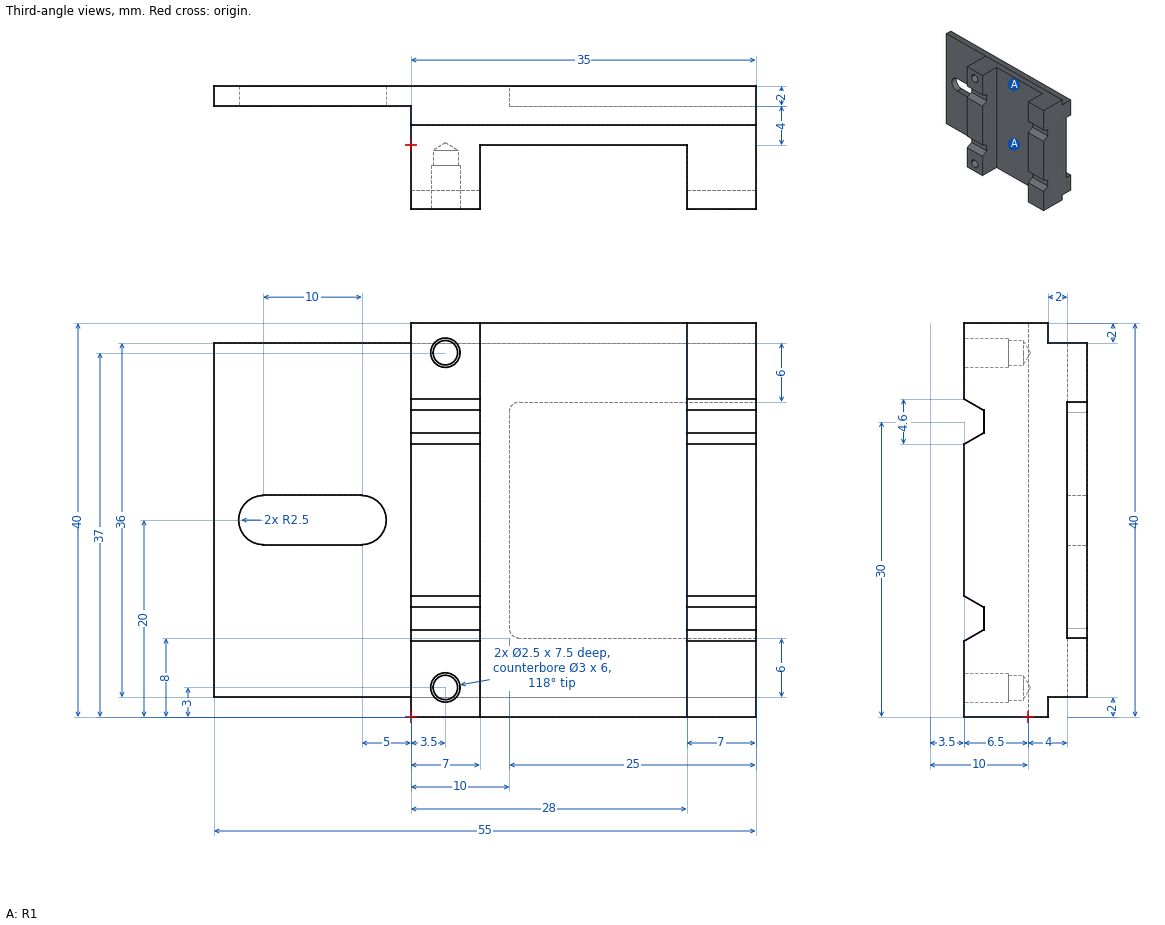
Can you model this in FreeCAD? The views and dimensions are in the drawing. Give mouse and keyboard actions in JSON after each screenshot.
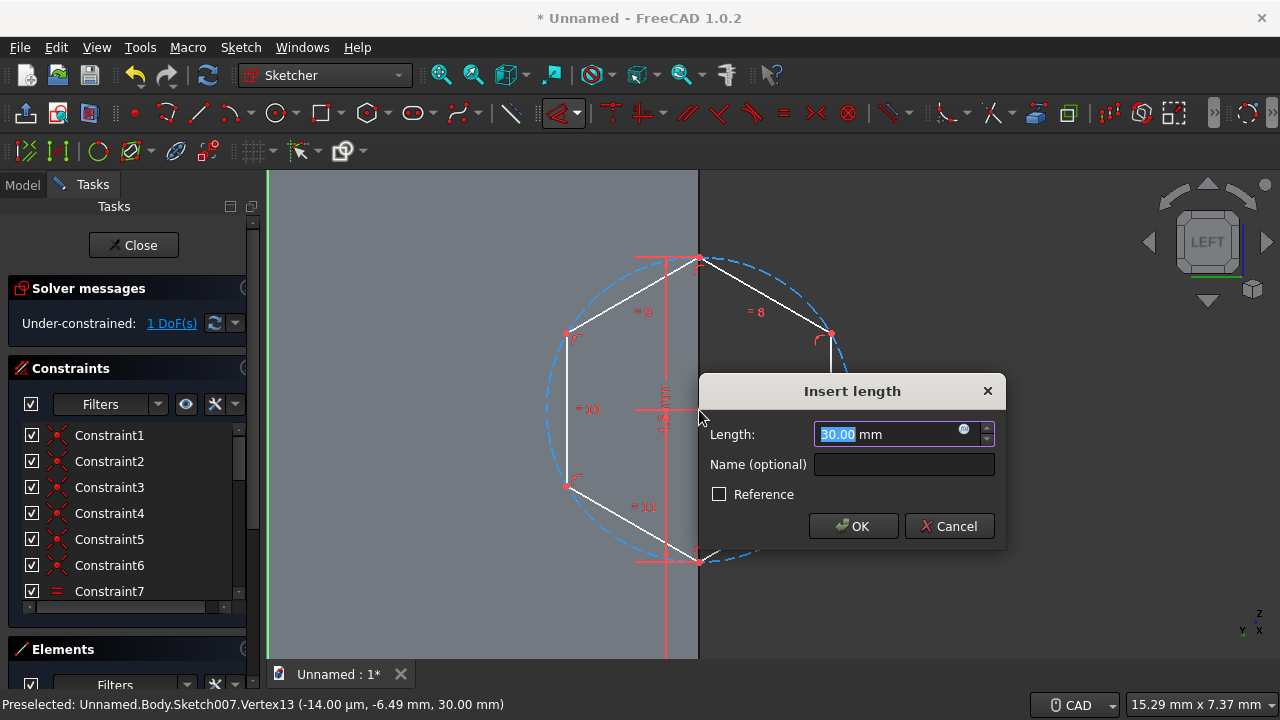
{"action": "type", "text": "30"}
{"action": "key", "text": "Return"}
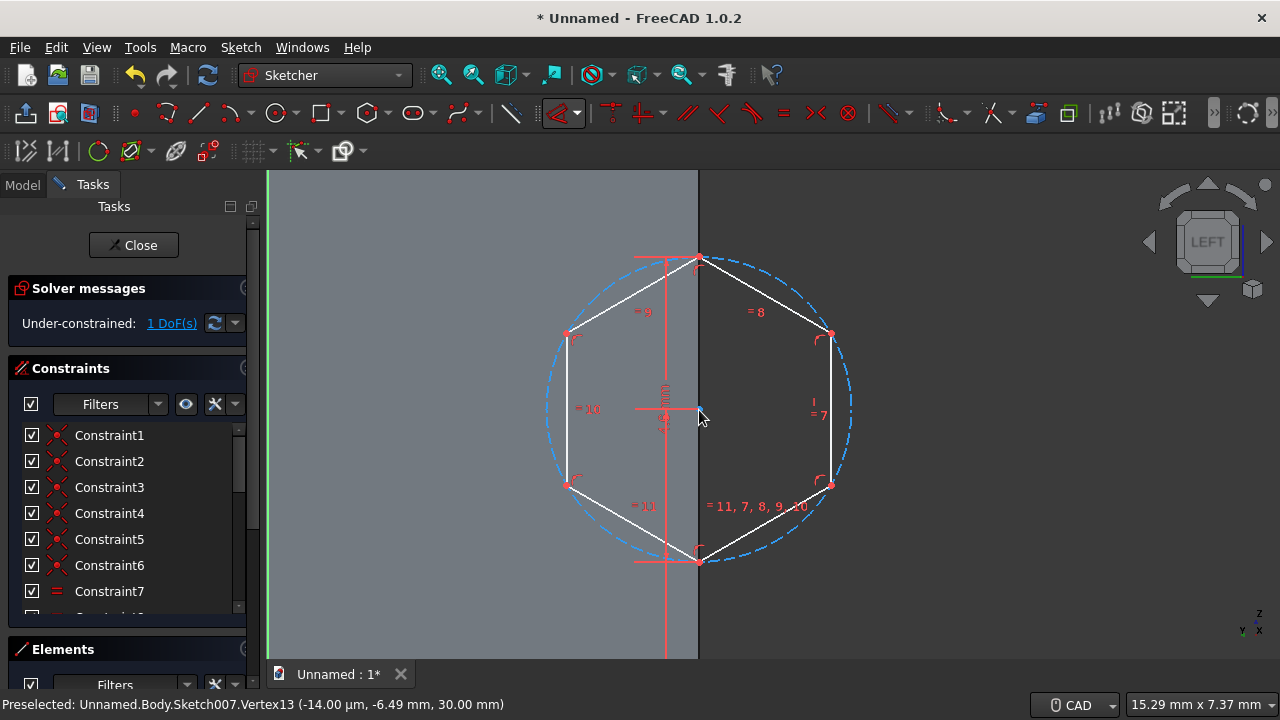
{"action": "left_click", "coordinate": [699, 409]}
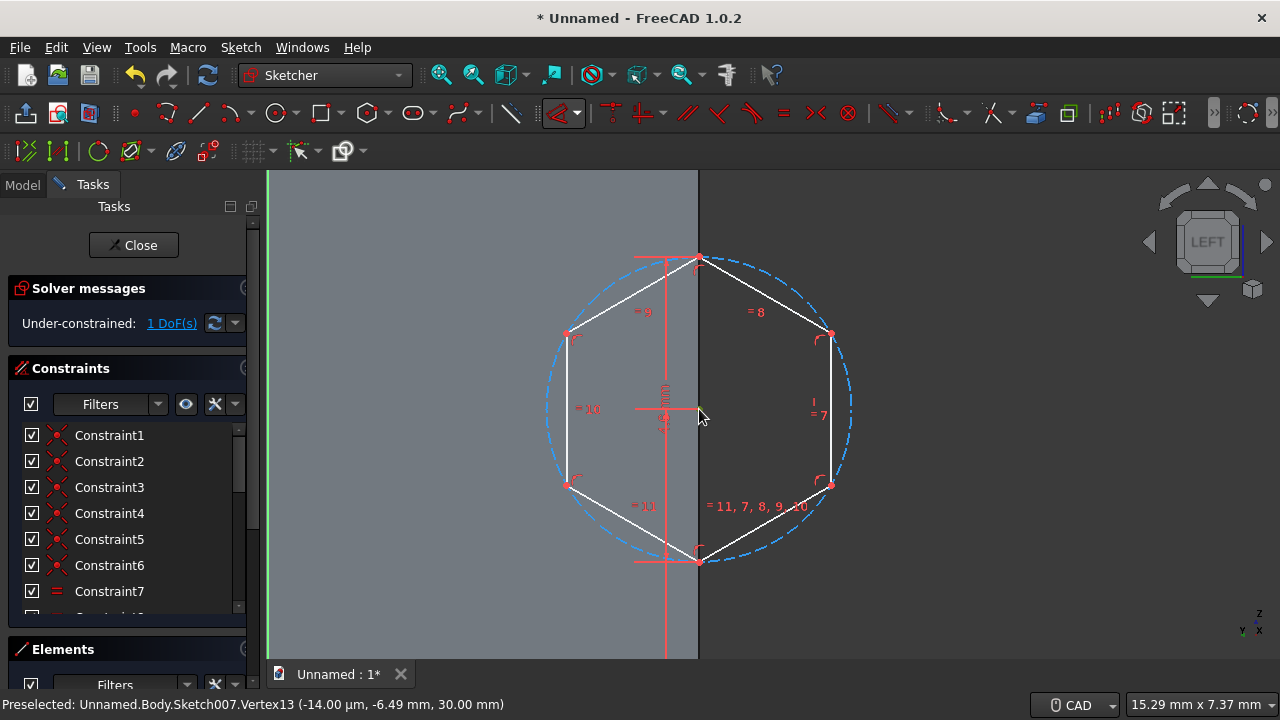
{"action": "key", "text": "l"}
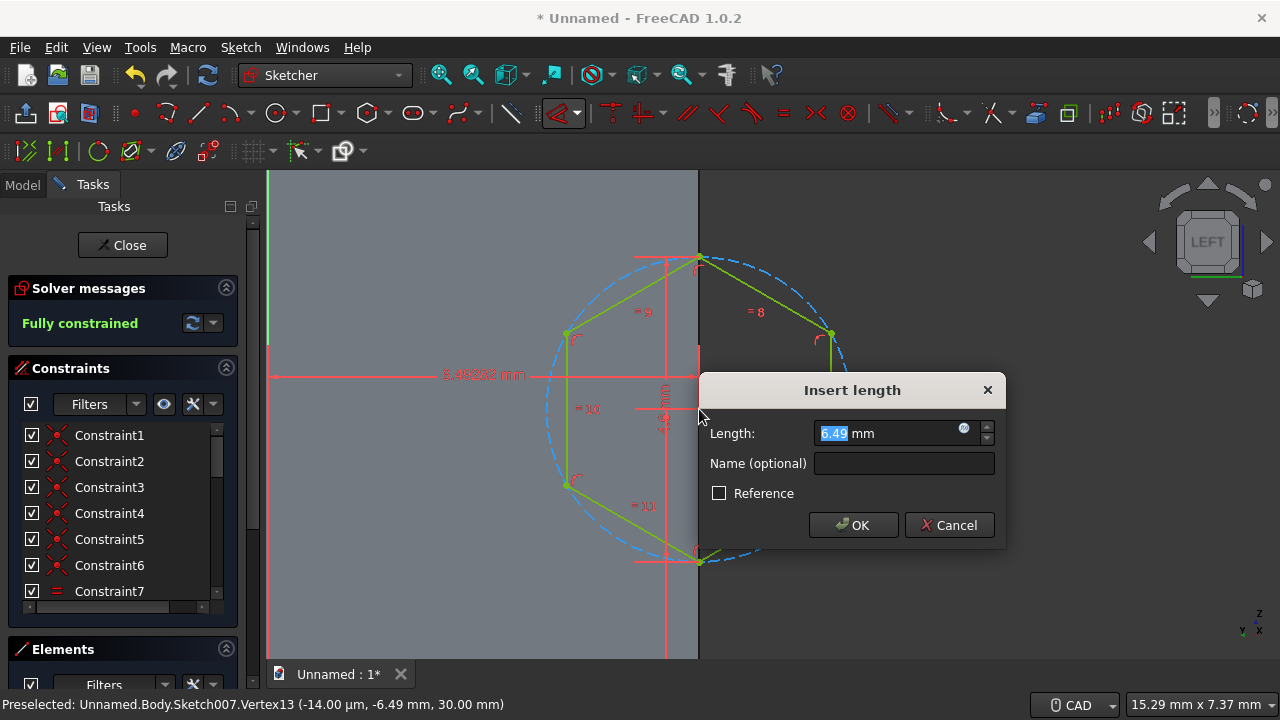
{"action": "type", "text": "6.5"}
{"action": "key", "text": "Return"}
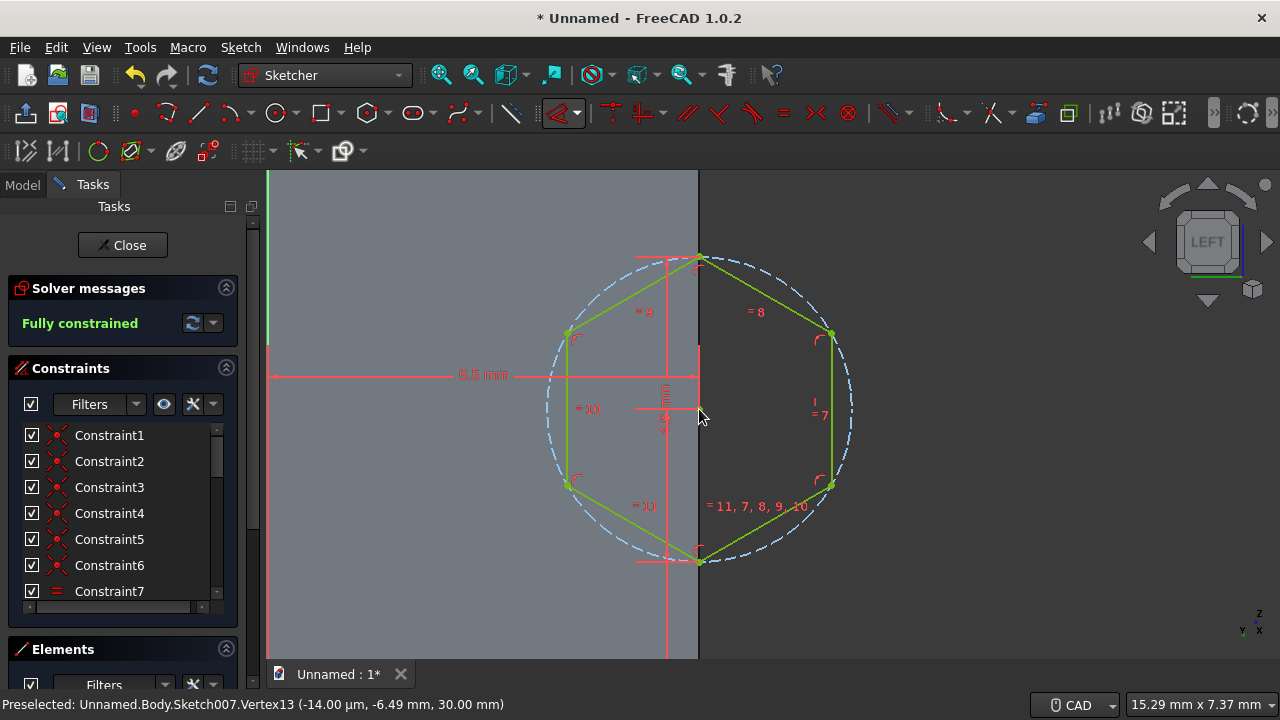
{"action": "left_click", "coordinate": [123, 245]}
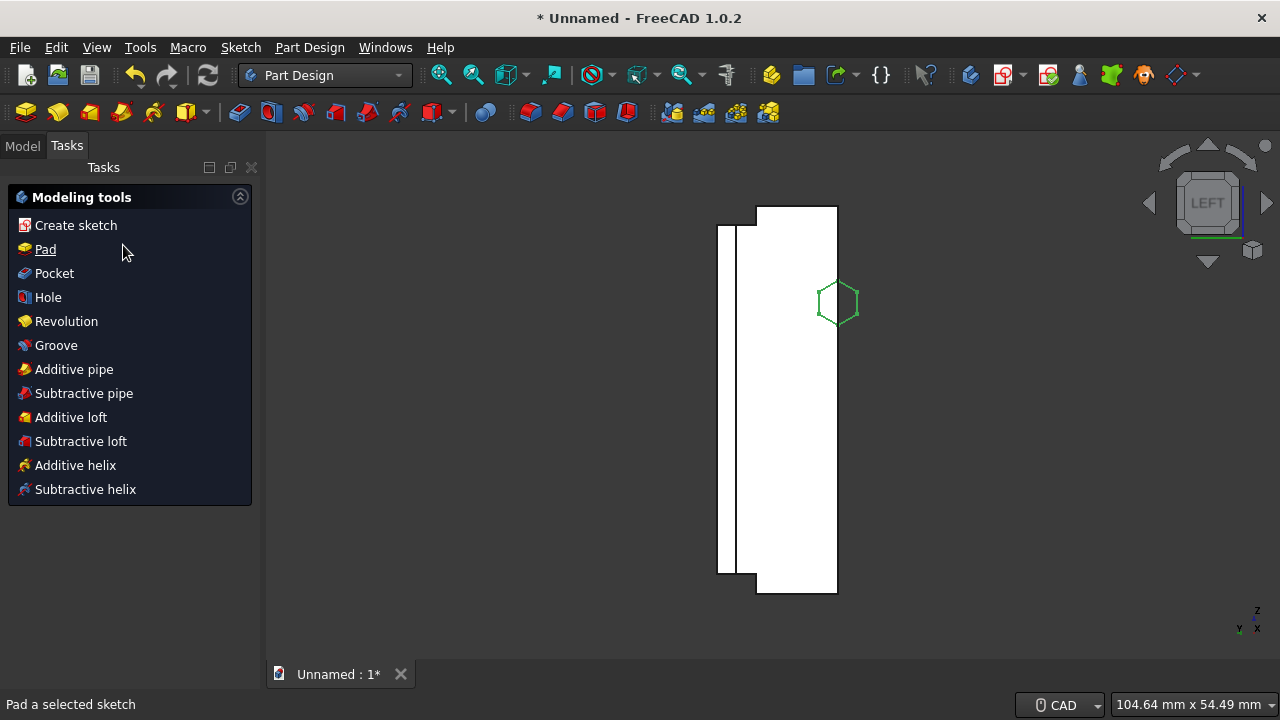
{"action": "left_click", "coordinate": [240, 112]}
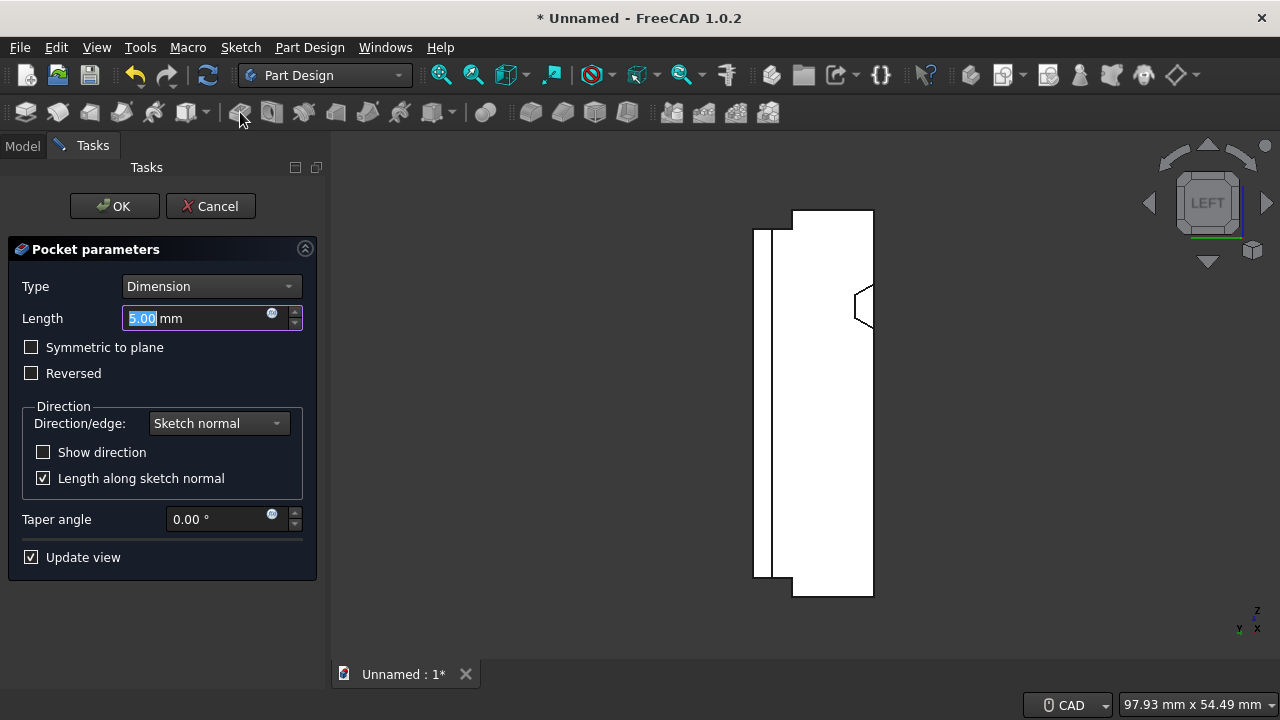
{"action": "left_click", "coordinate": [212, 286]}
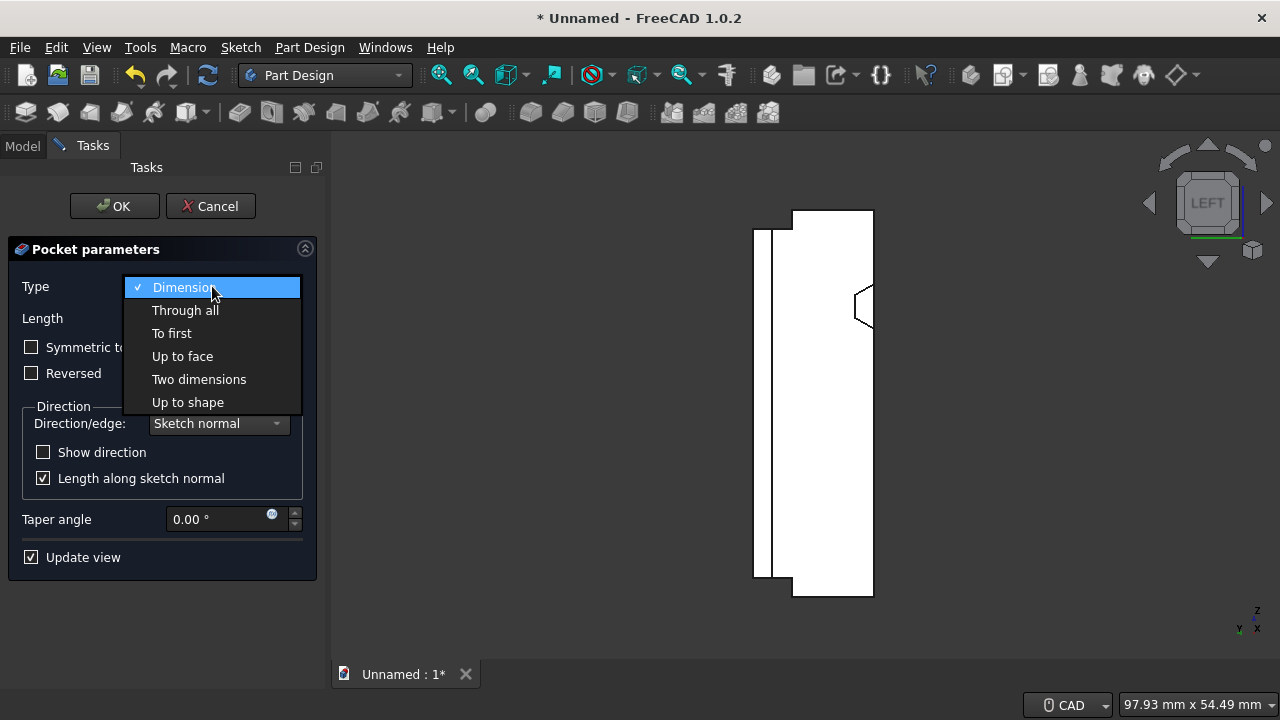
{"action": "left_click", "coordinate": [212, 310]}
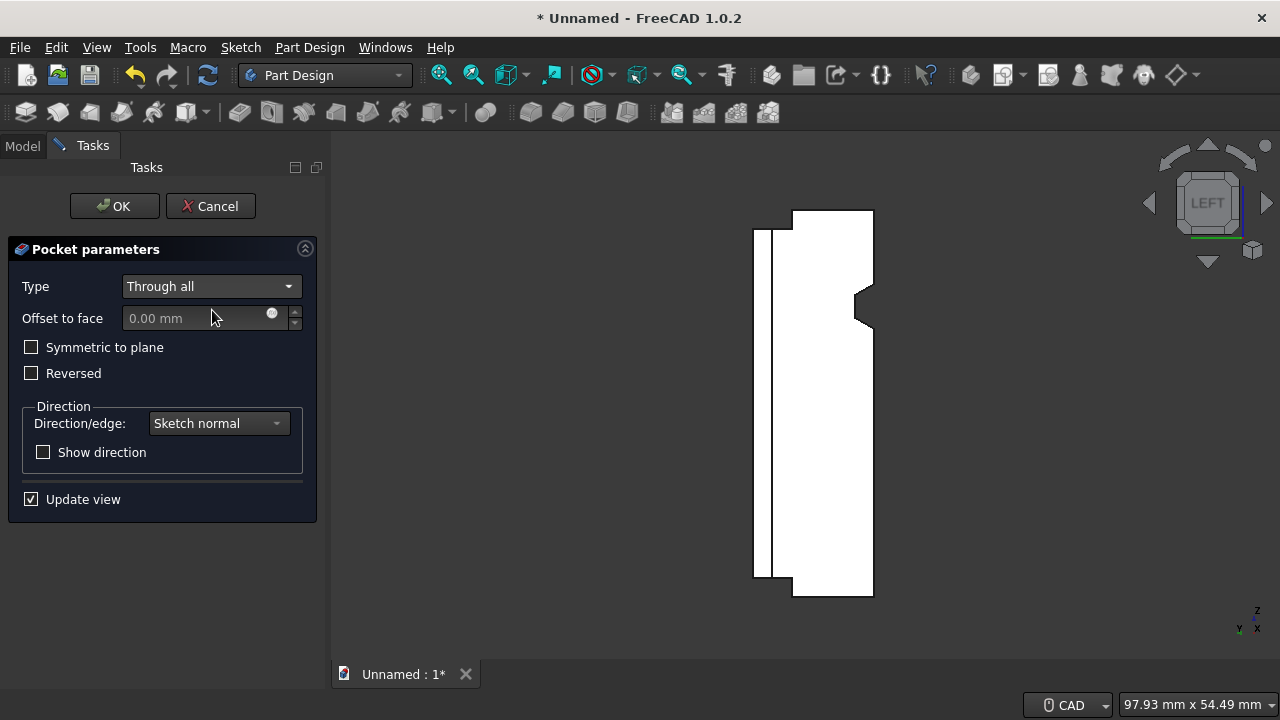
{"action": "left_click", "coordinate": [115, 206]}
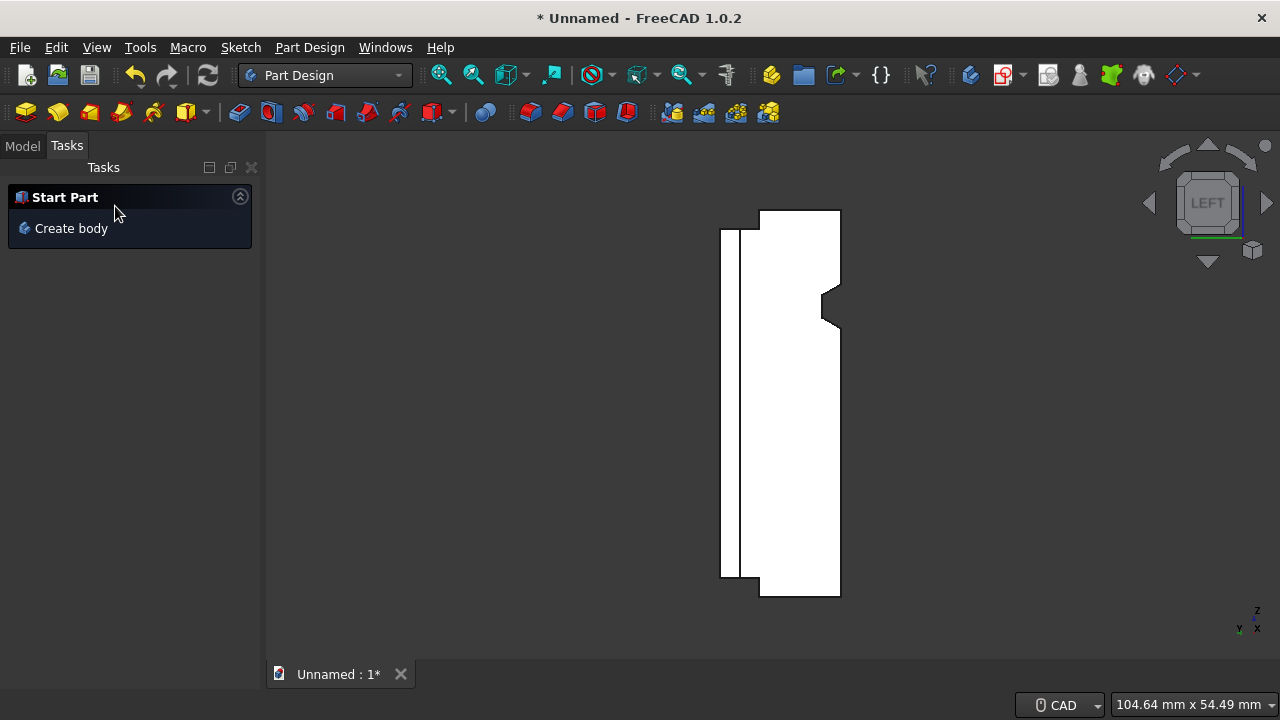
{"action": "left_click", "coordinate": [23, 145]}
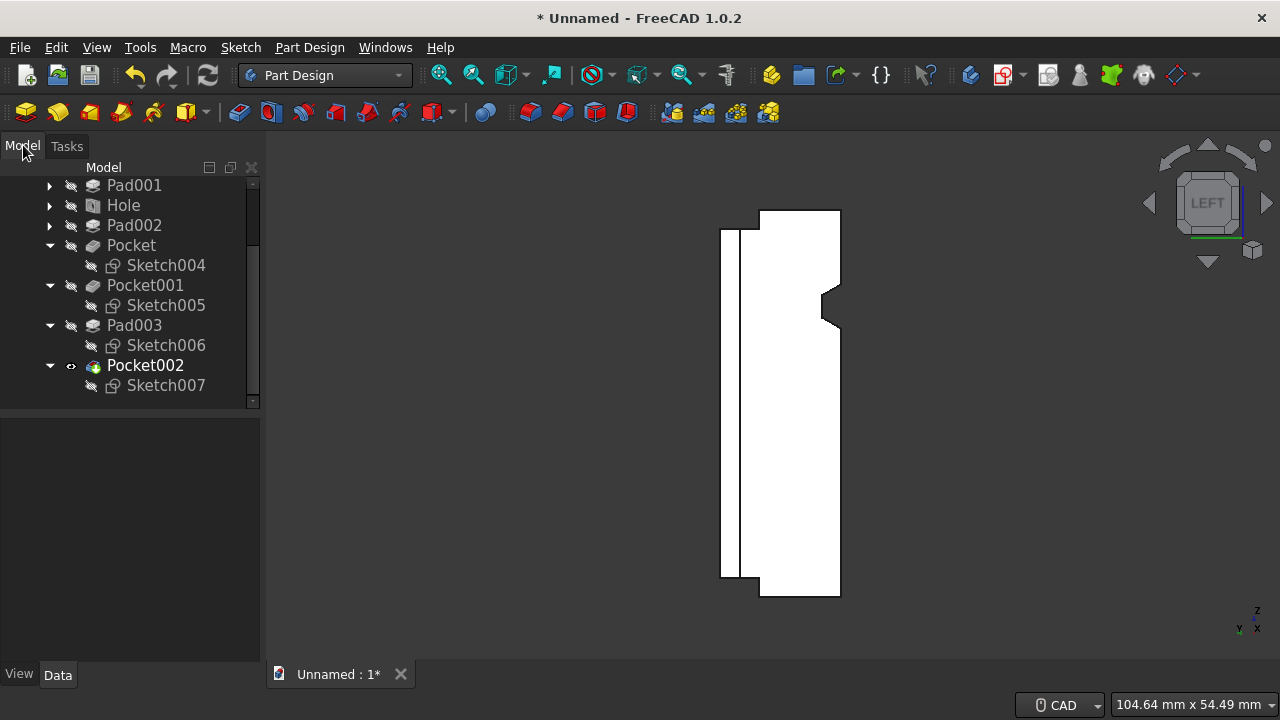
{"action": "scroll", "coordinate": [140, 281], "scroll_direction": "down", "scroll_amount": 3}